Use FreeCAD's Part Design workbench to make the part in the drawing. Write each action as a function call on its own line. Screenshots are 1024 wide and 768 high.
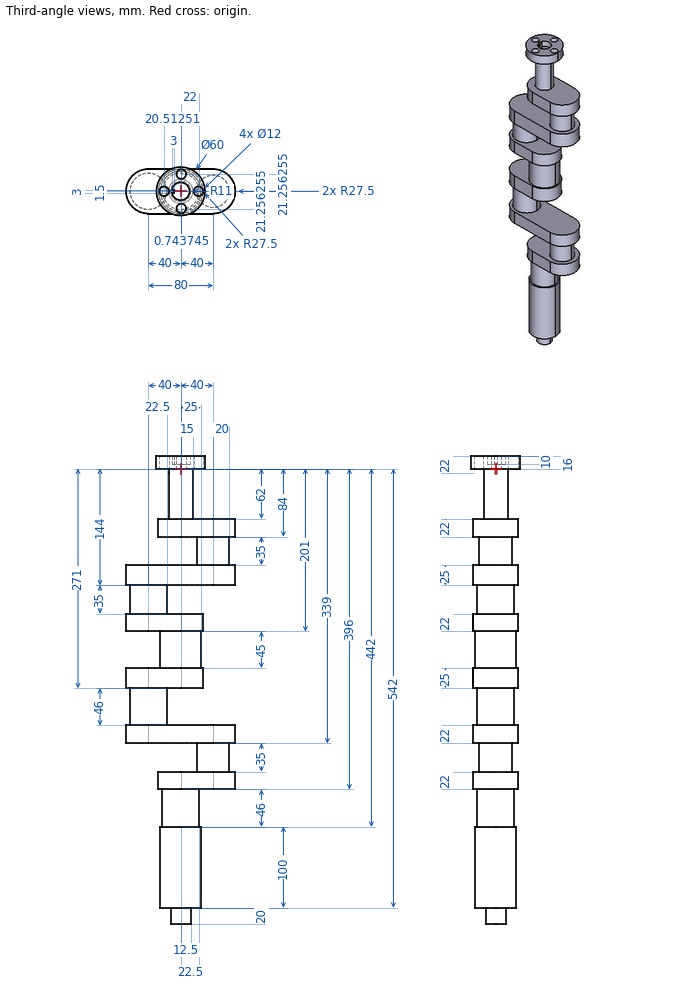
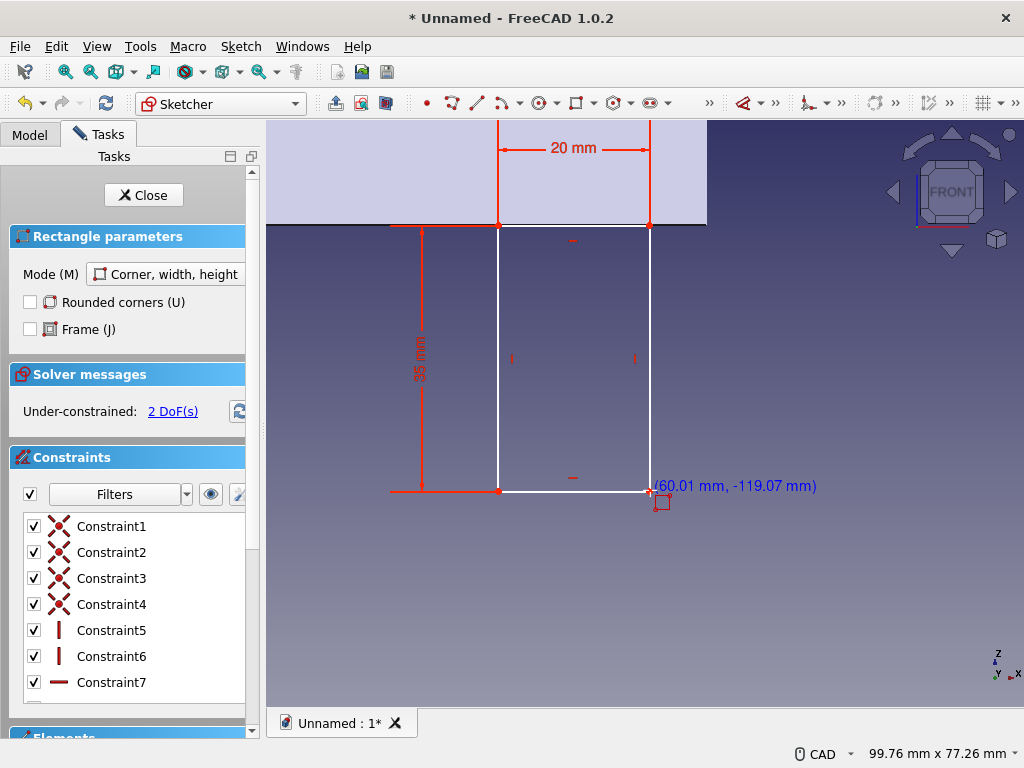
click(477, 104)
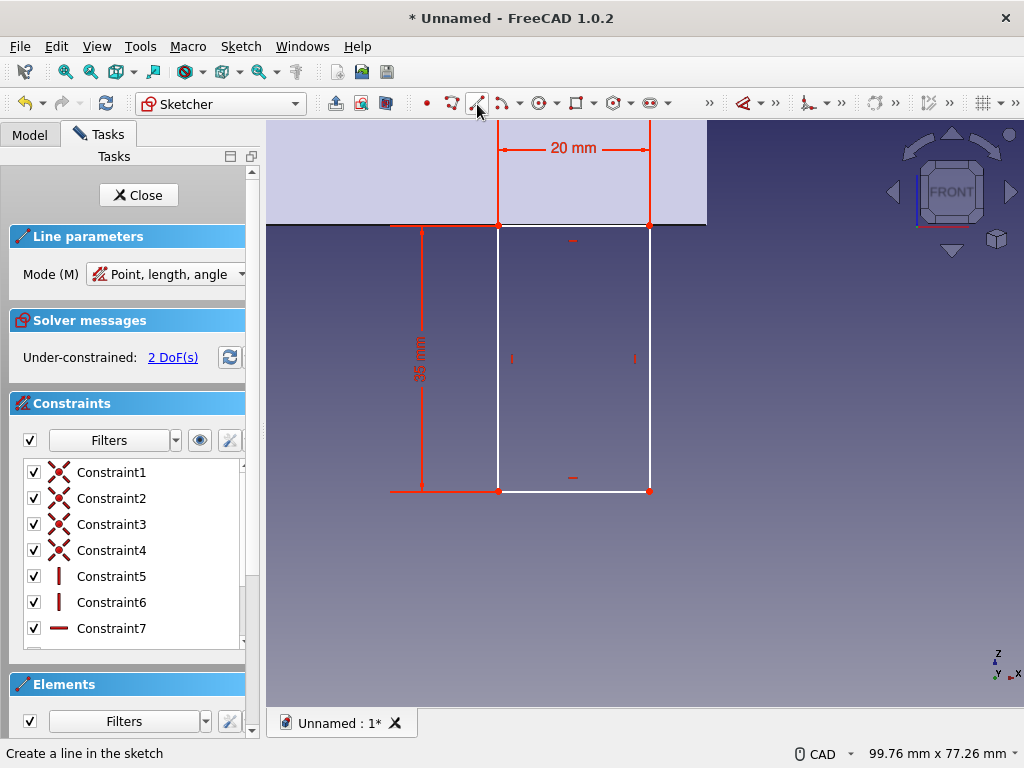
click(498, 517)
click(498, 597)
key(Escape)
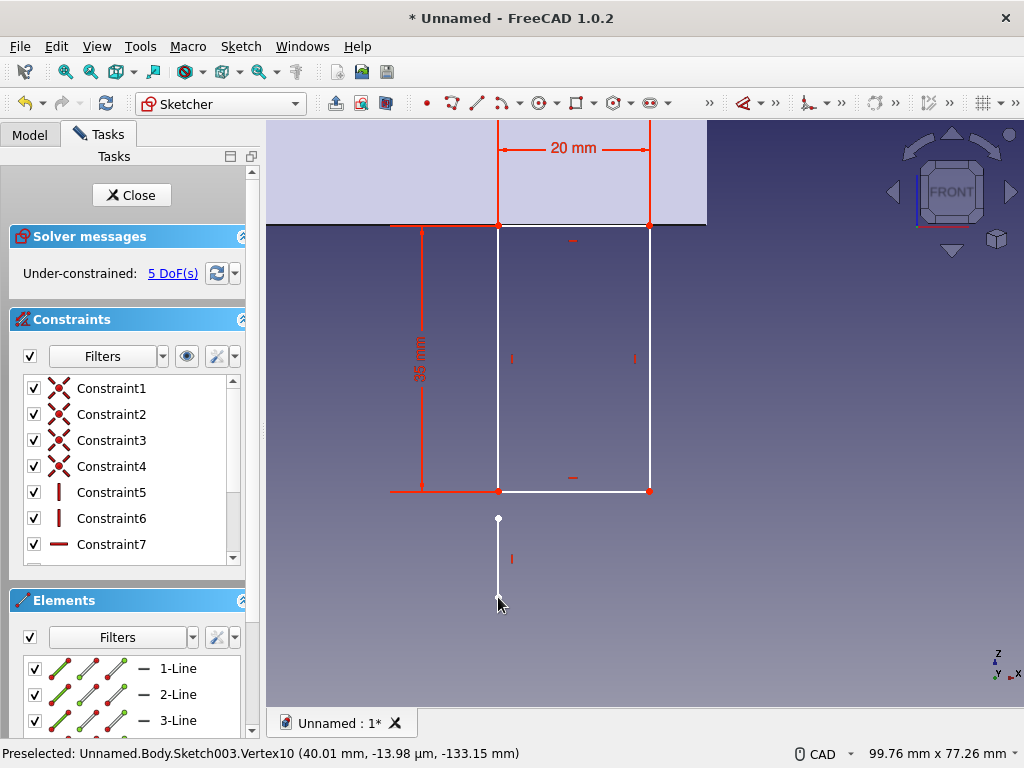
click(498, 542)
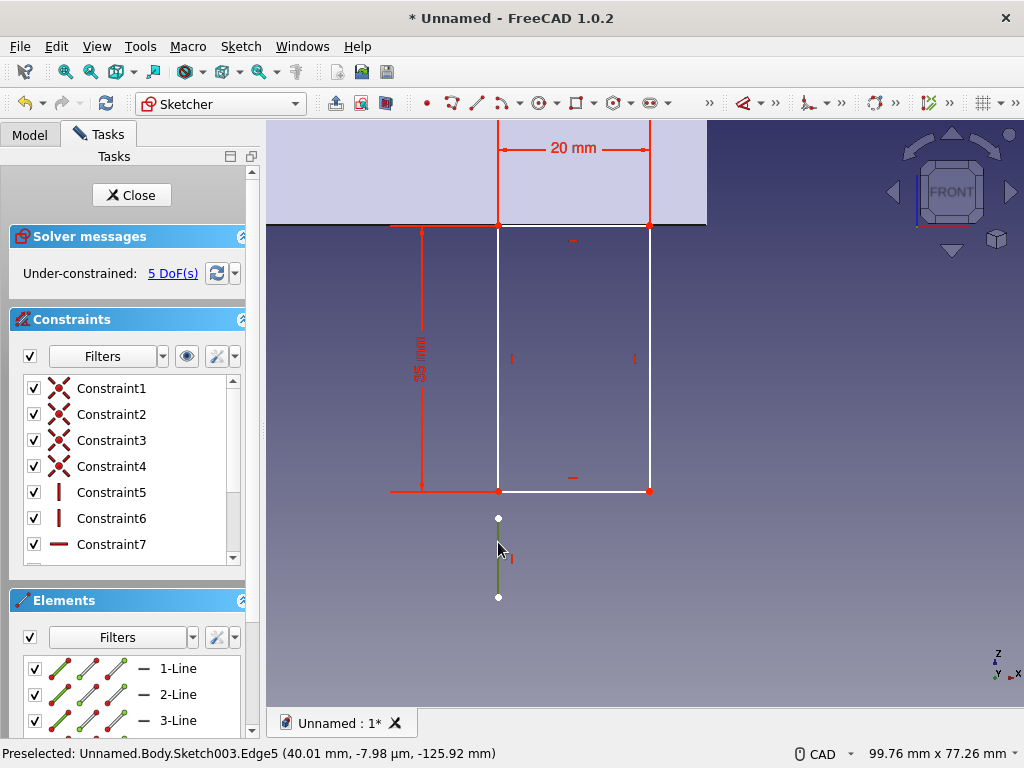
key(g)
key(n)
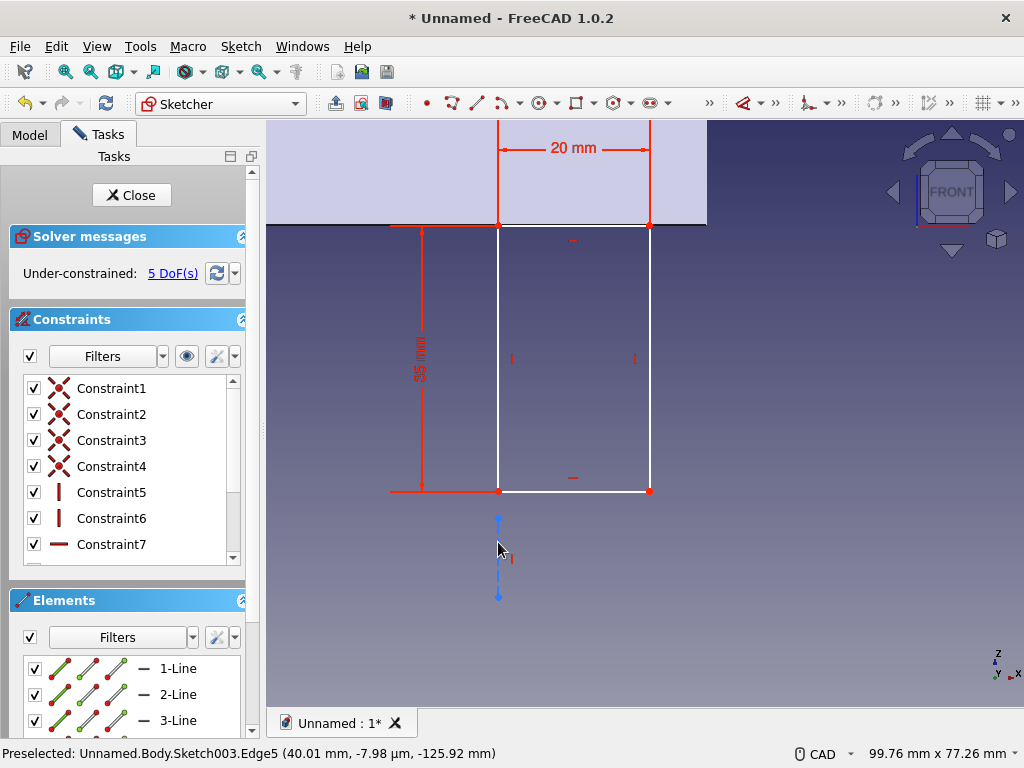
click(742, 104)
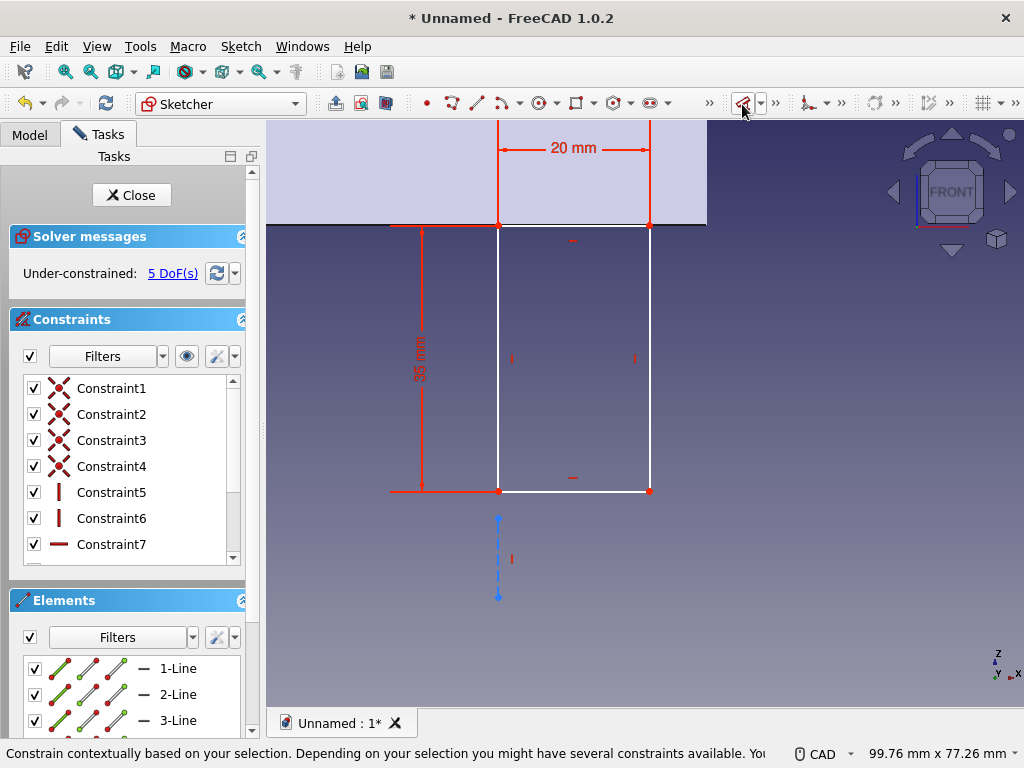
click(498, 226)
click(396, 260)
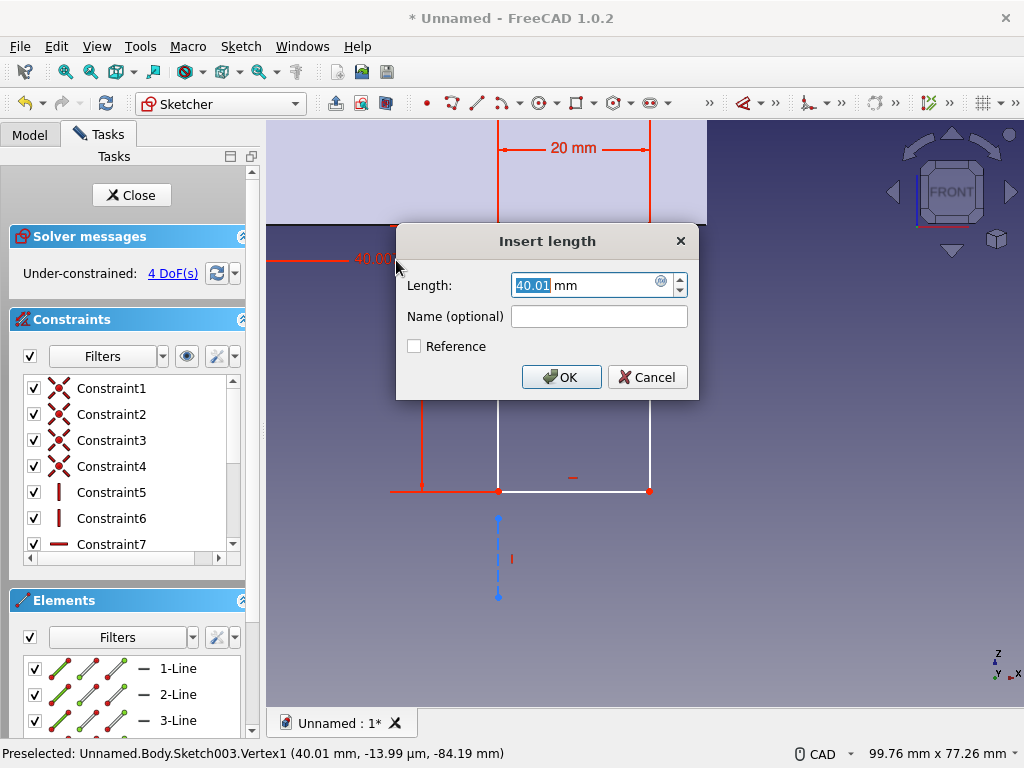
text(40)
key(Return)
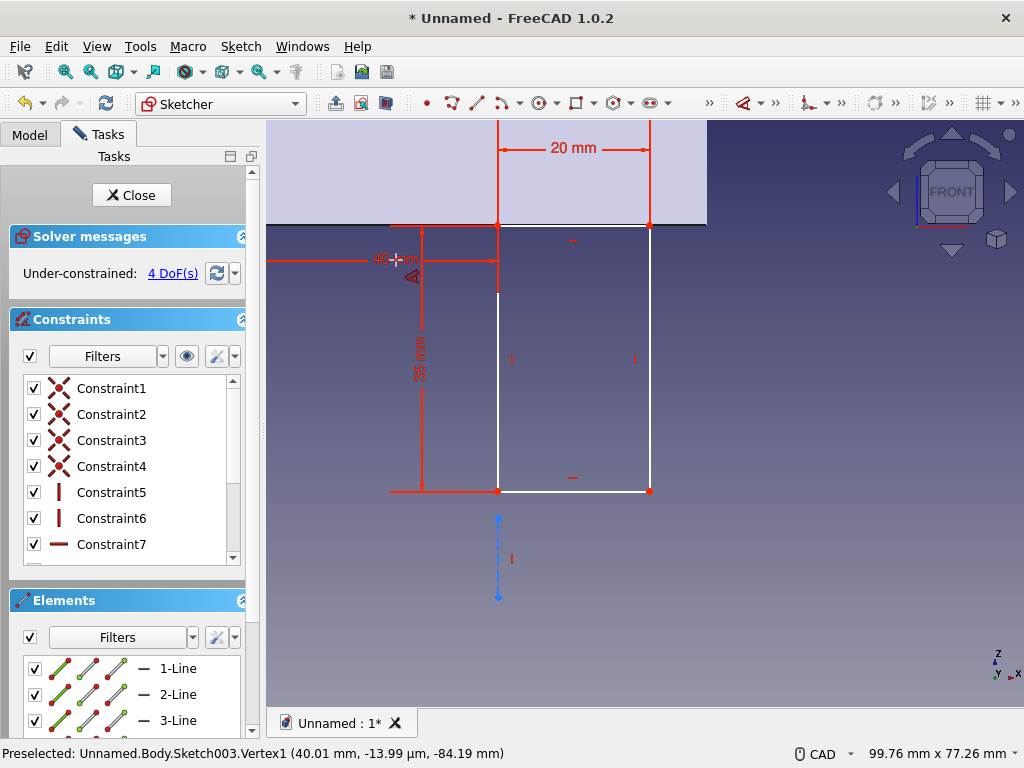
click(498, 226)
click(532, 187)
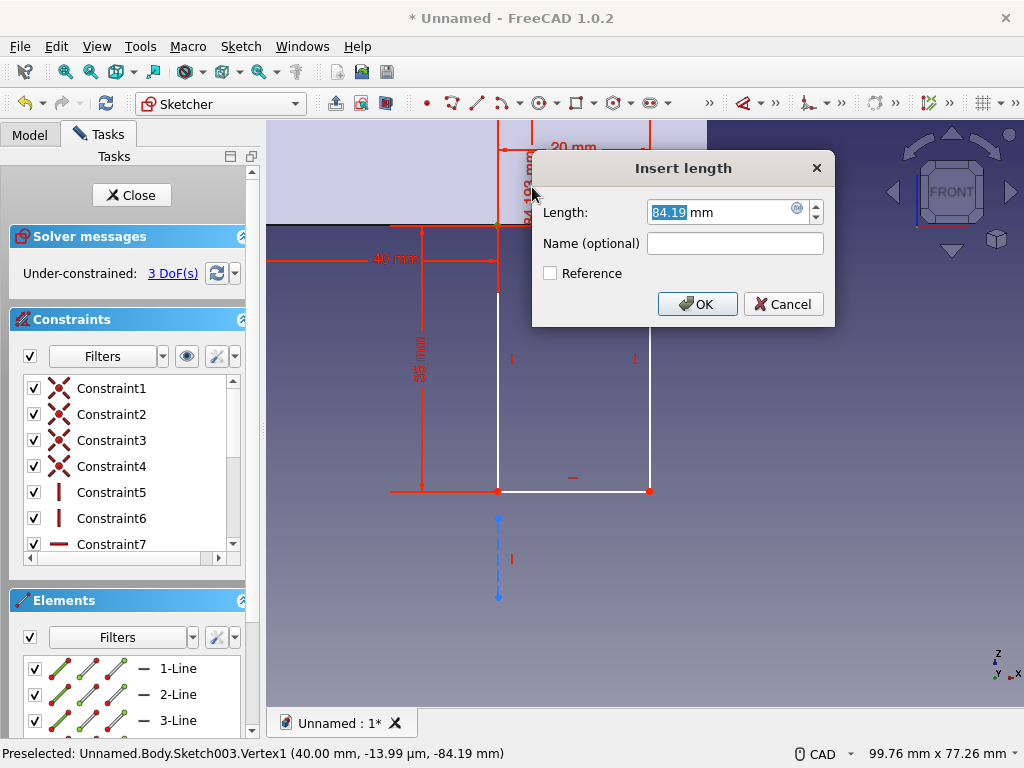
text(84)
key(Return)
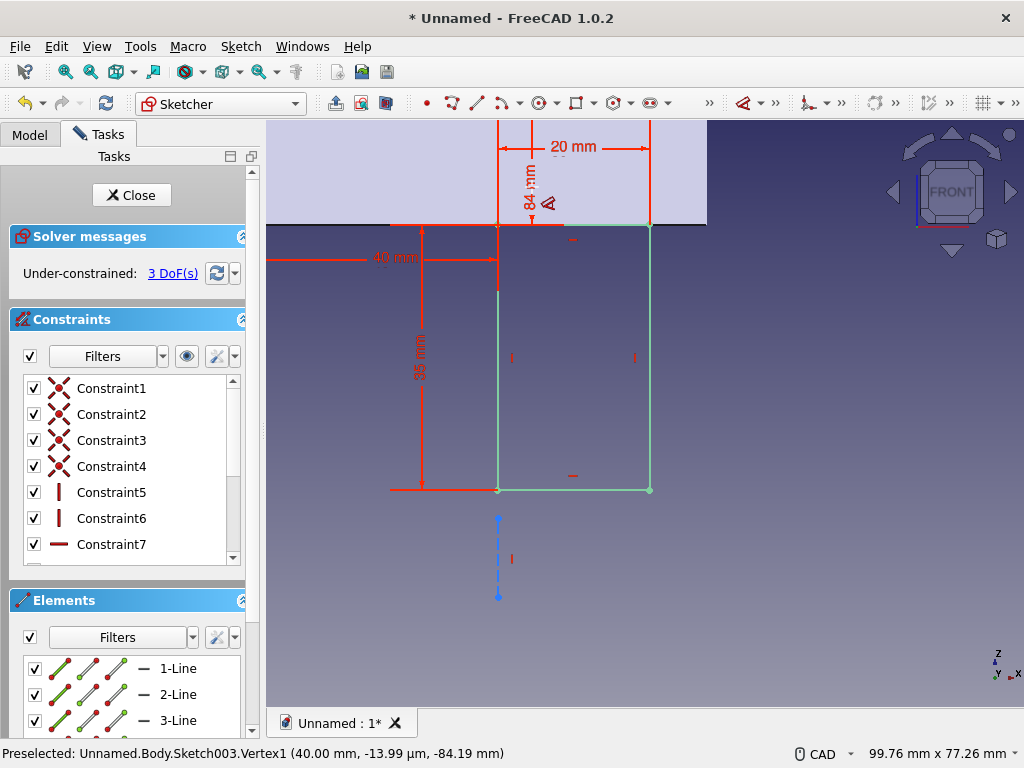
click(498, 518)
click(396, 552)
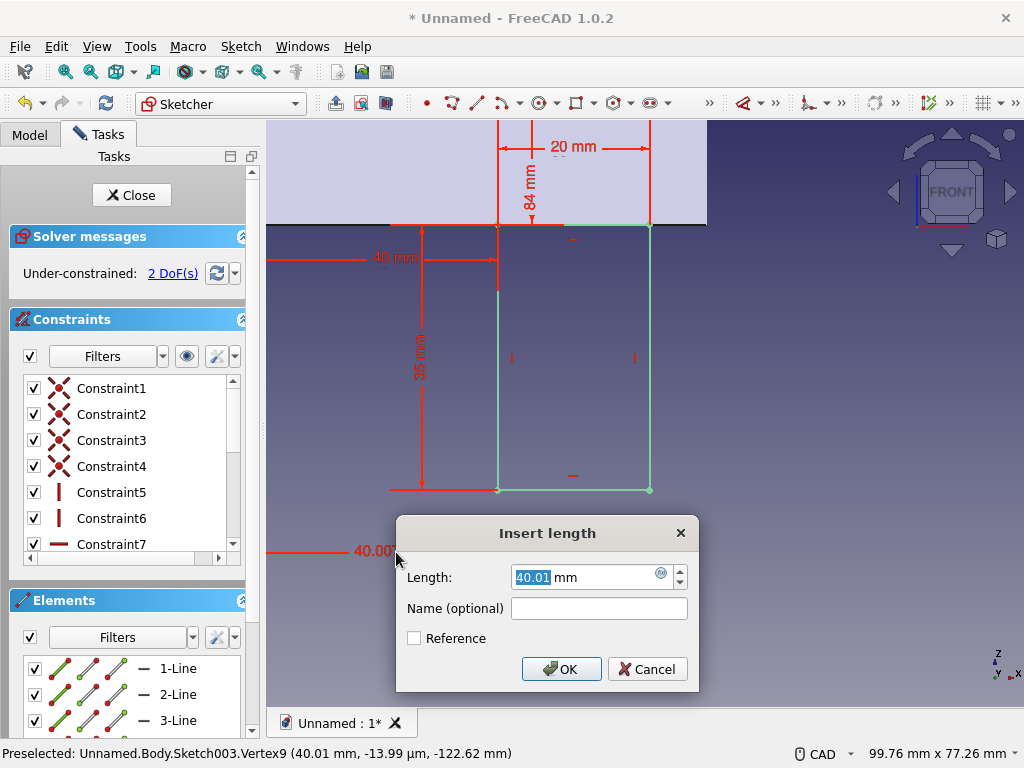
text(40)
key(Return)
key(Escape)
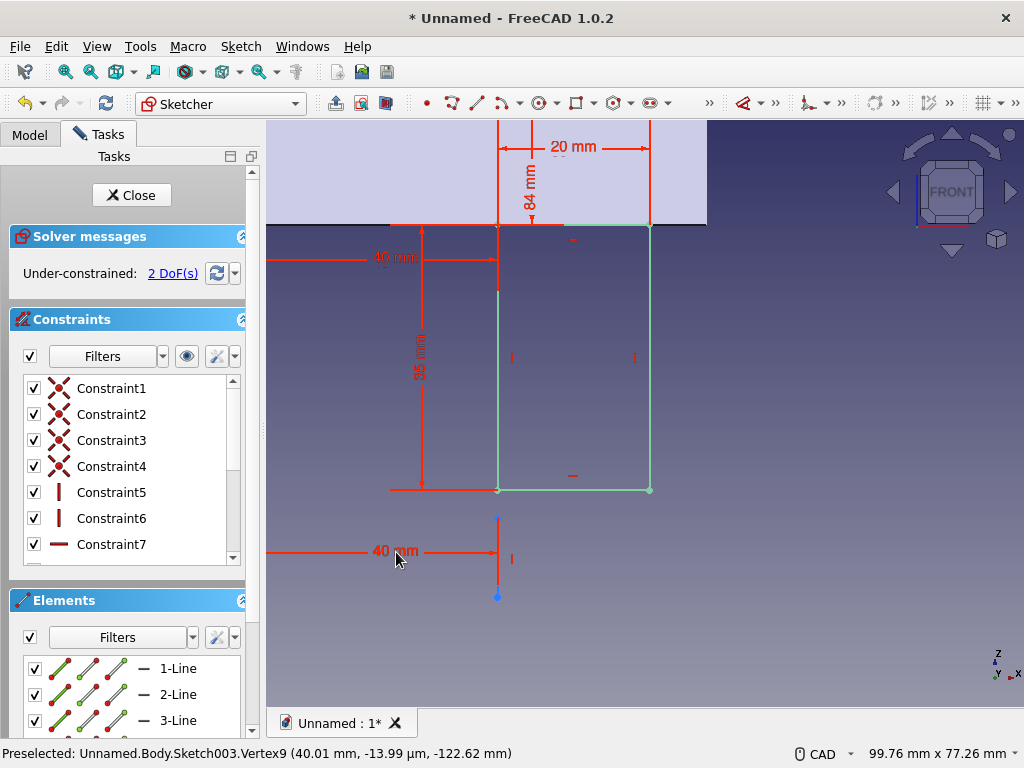
click(132, 195)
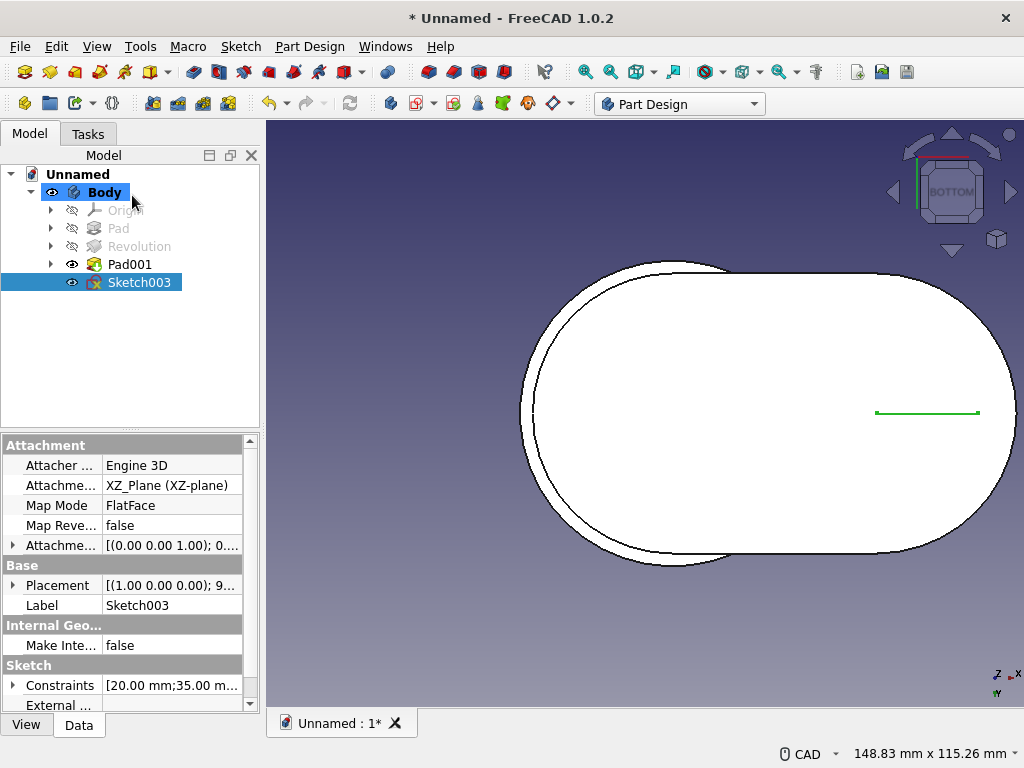
click(50, 72)